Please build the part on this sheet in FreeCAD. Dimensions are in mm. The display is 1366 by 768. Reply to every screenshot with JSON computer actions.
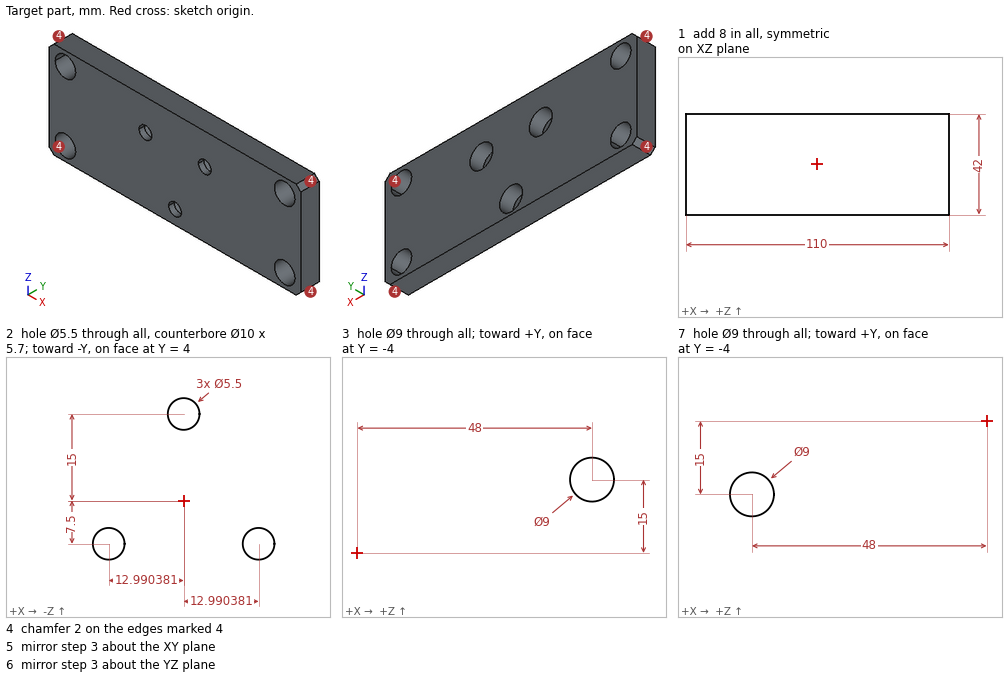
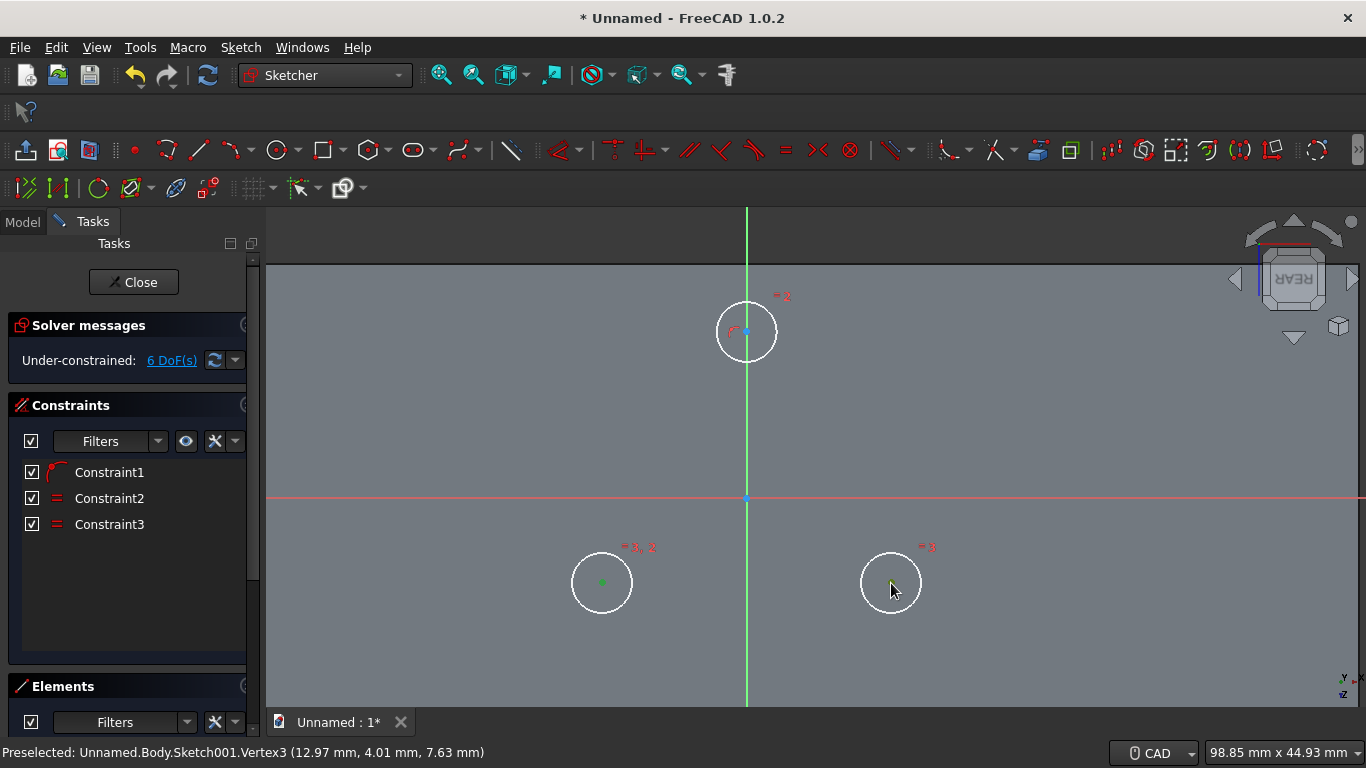
{"action": "left_click", "coordinate": [668, 150]}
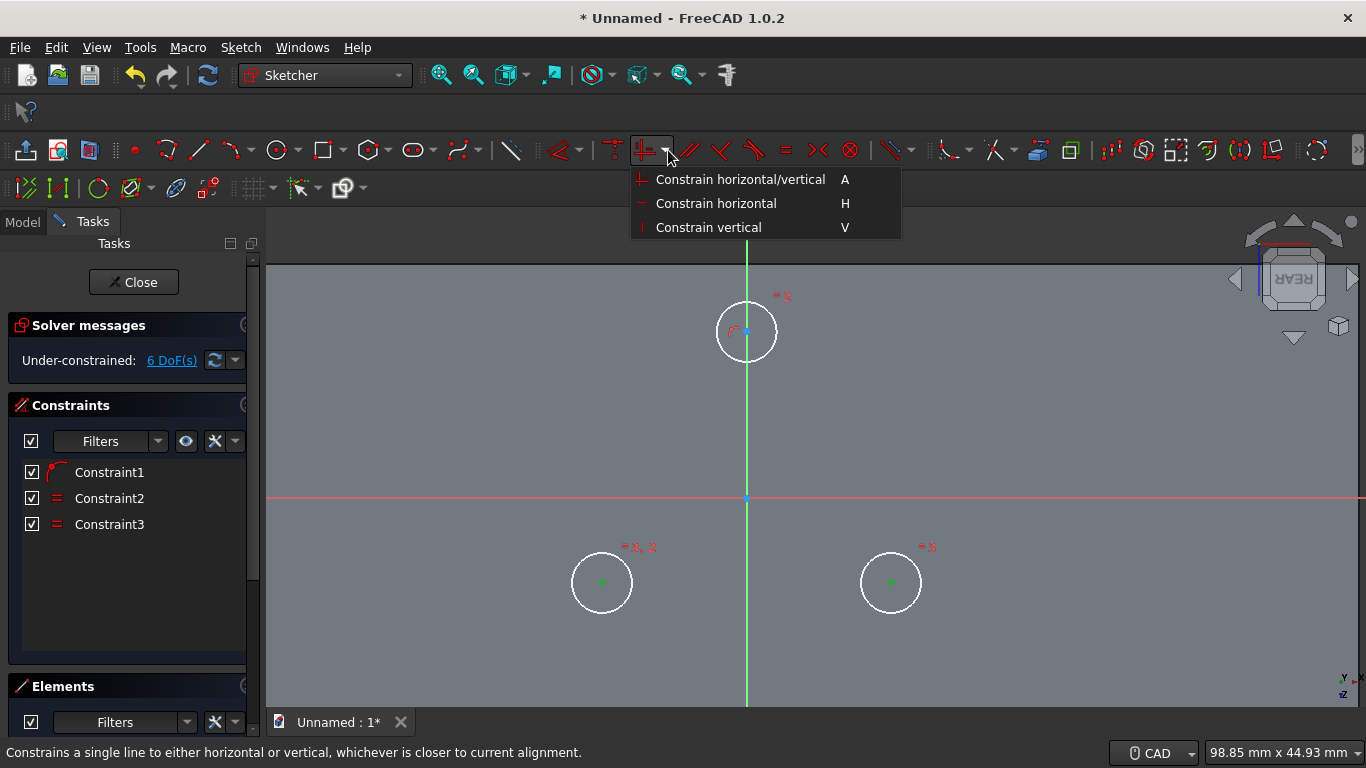
{"action": "left_click", "coordinate": [766, 203]}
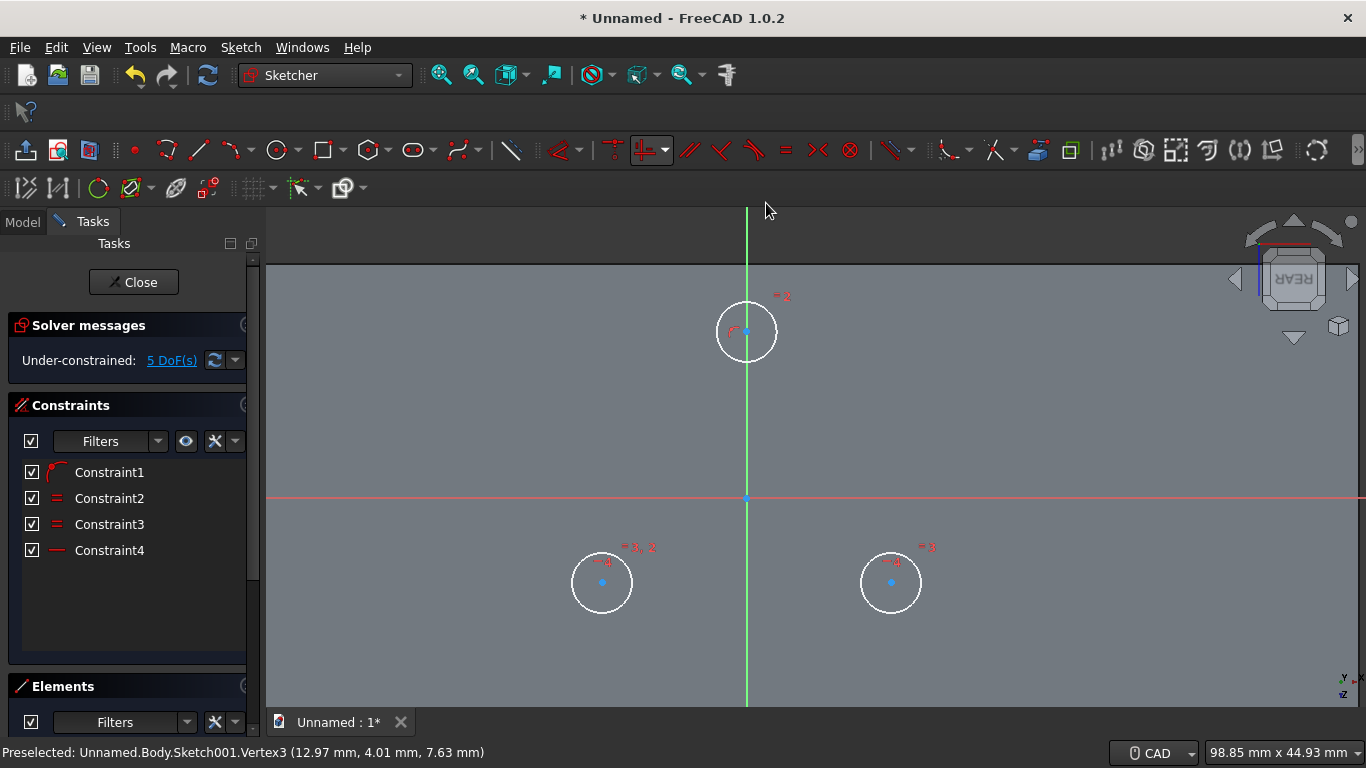
{"action": "left_click", "coordinate": [558, 150]}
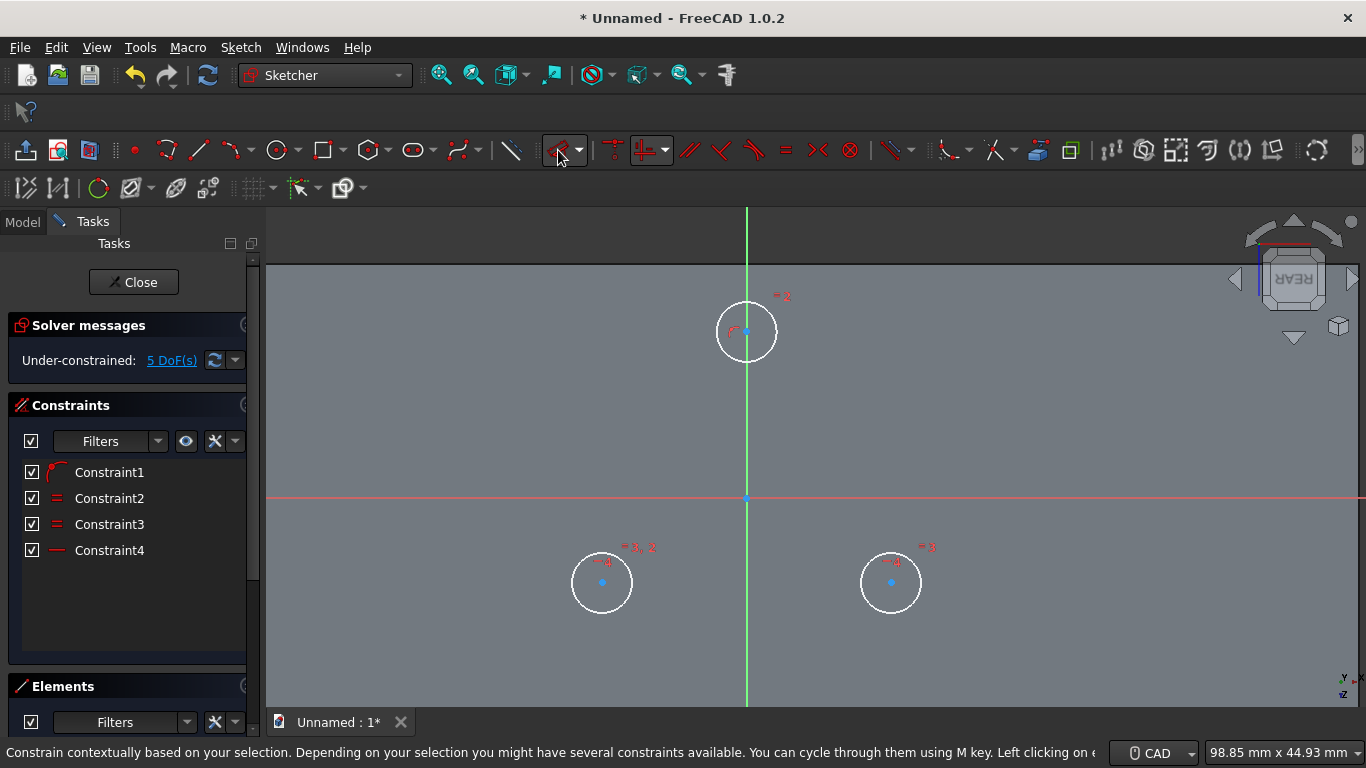
{"action": "left_click", "coordinate": [768, 311]}
{"action": "left_click", "coordinate": [791, 289]}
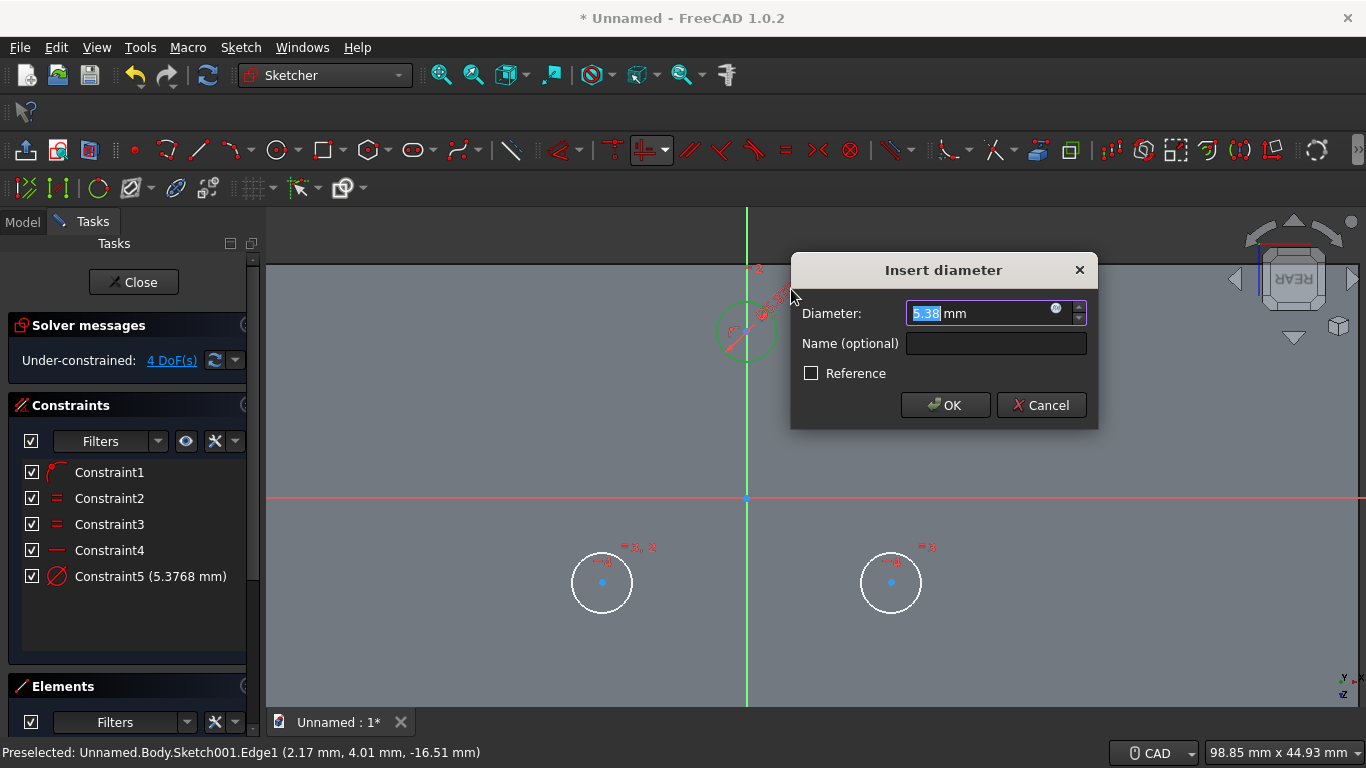
{"action": "type", "text": "5.5"}
{"action": "key", "text": "Return"}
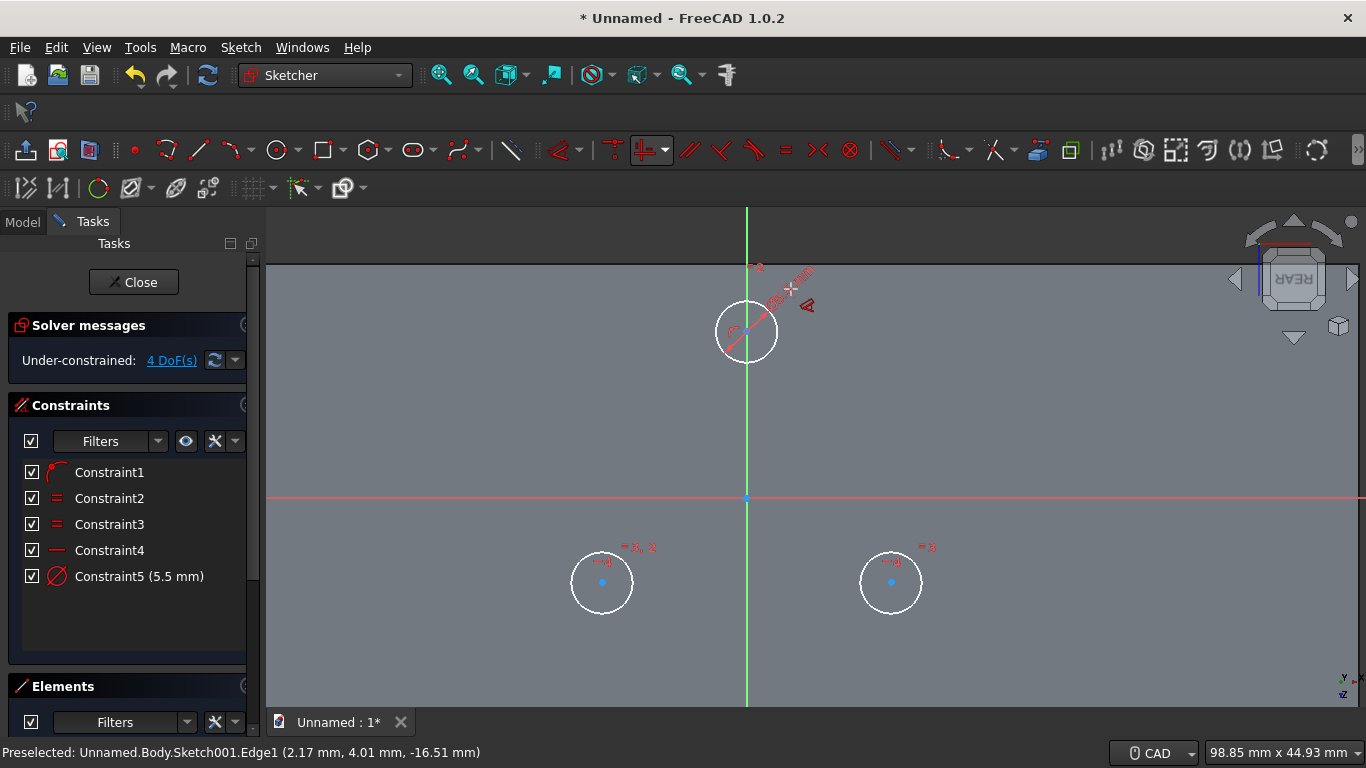
{"action": "left_click", "coordinate": [747, 332]}
{"action": "left_click", "coordinate": [781, 415]}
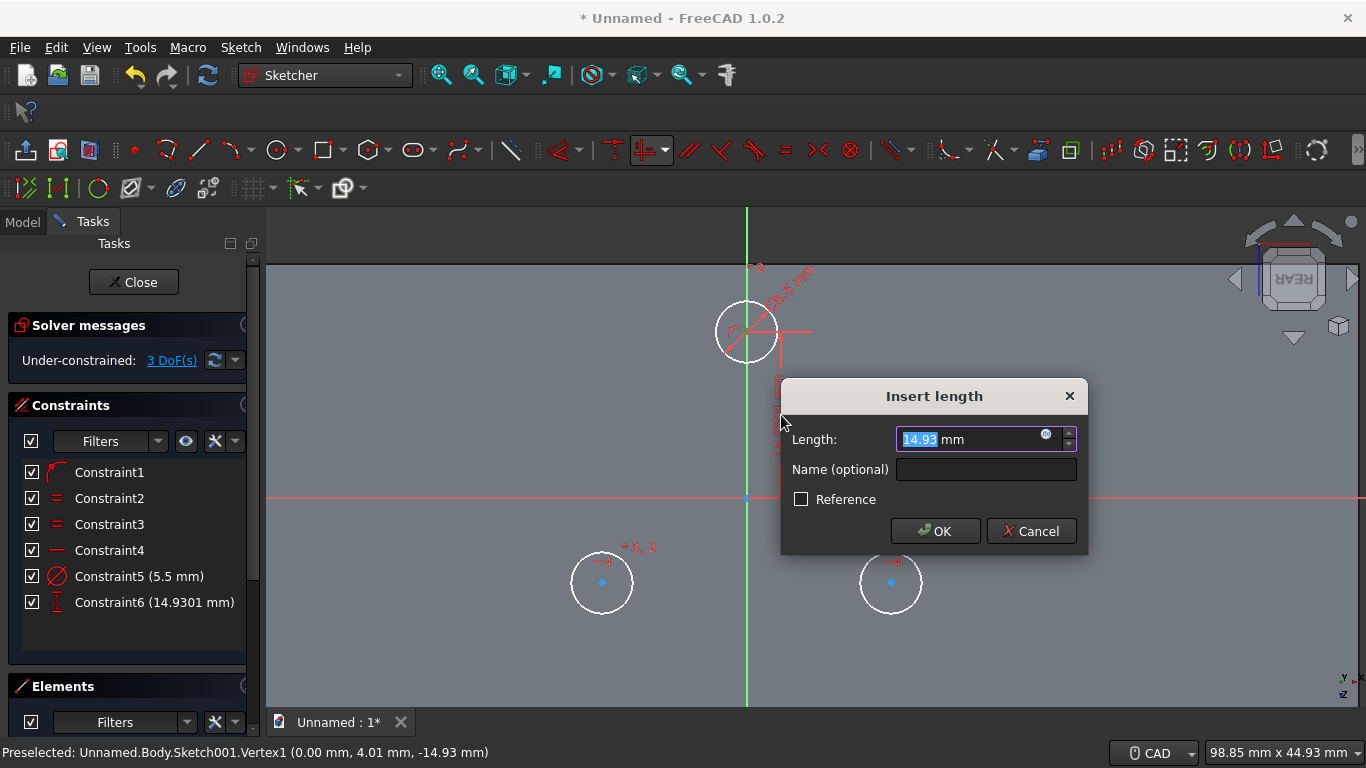
{"action": "type", "text": "15"}
{"action": "key", "text": "Return"}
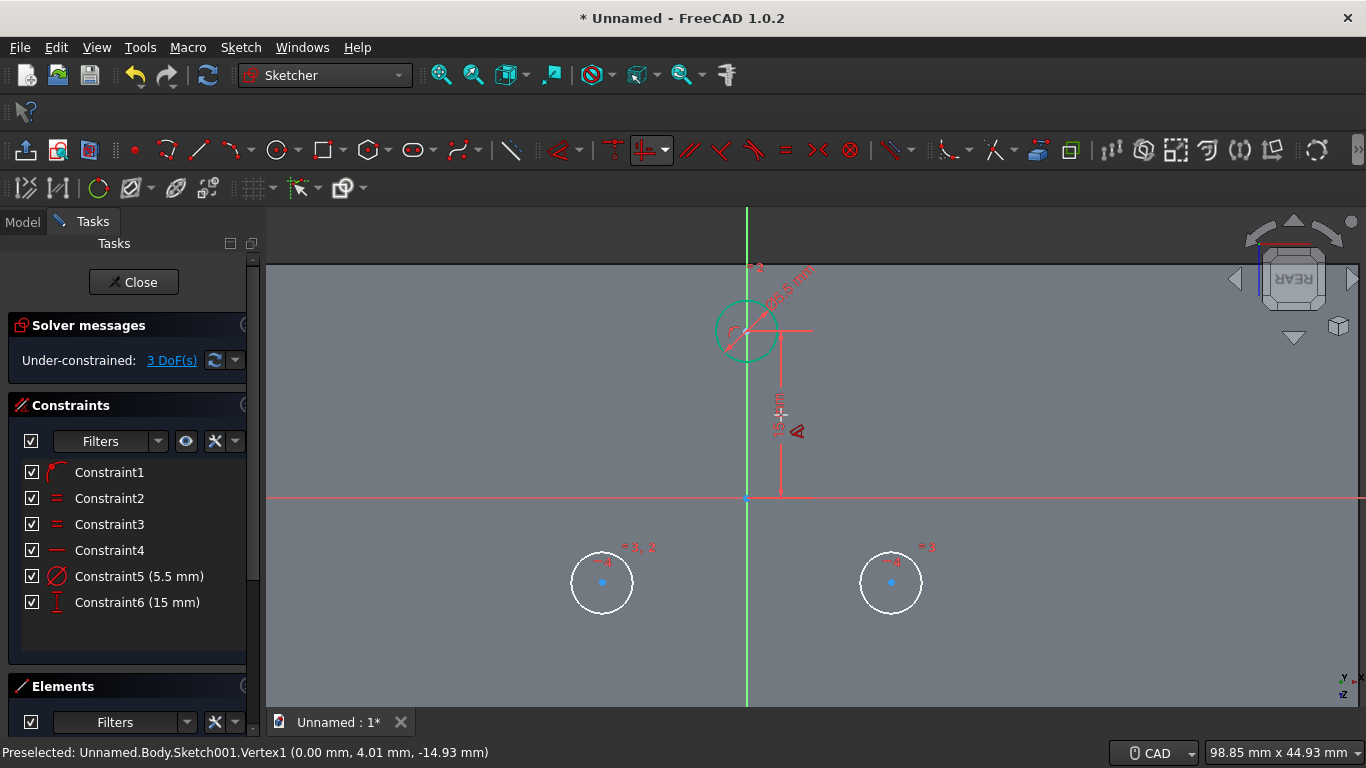
{"action": "left_click", "coordinate": [602, 583]}
{"action": "left_click", "coordinate": [568, 541]}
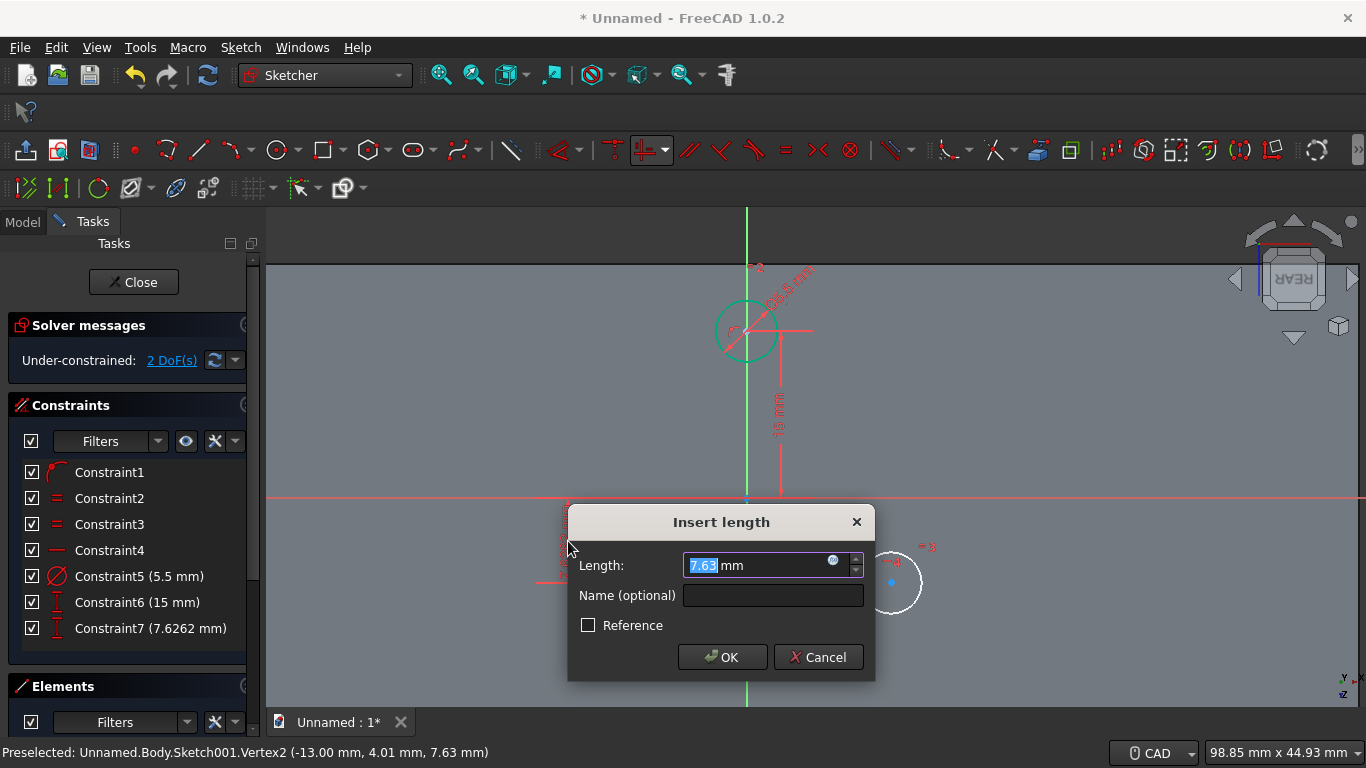
{"action": "type", "text": "7.5"}
{"action": "key", "text": "Return"}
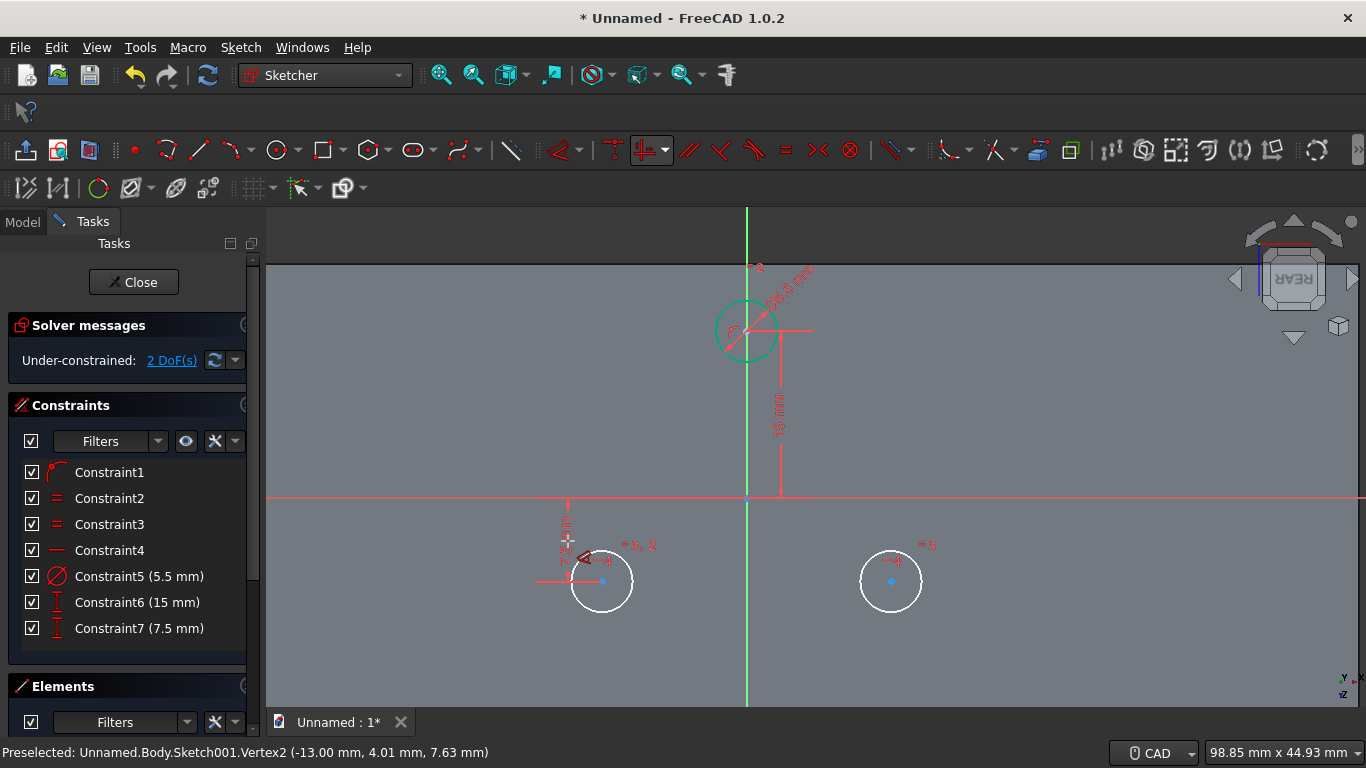
{"action": "left_click", "coordinate": [602, 582]}
{"action": "left_click", "coordinate": [674, 616]}